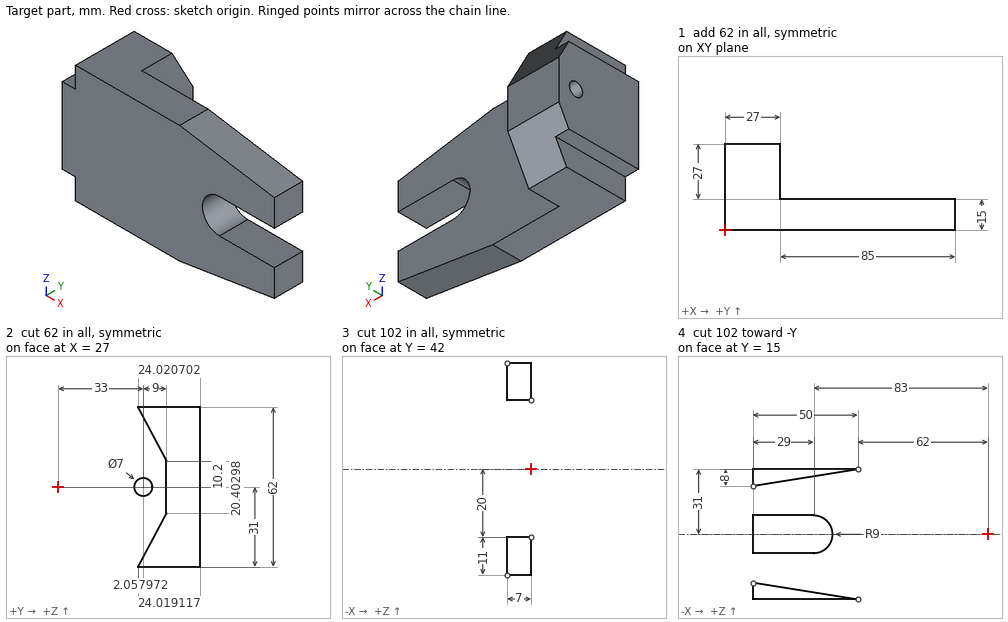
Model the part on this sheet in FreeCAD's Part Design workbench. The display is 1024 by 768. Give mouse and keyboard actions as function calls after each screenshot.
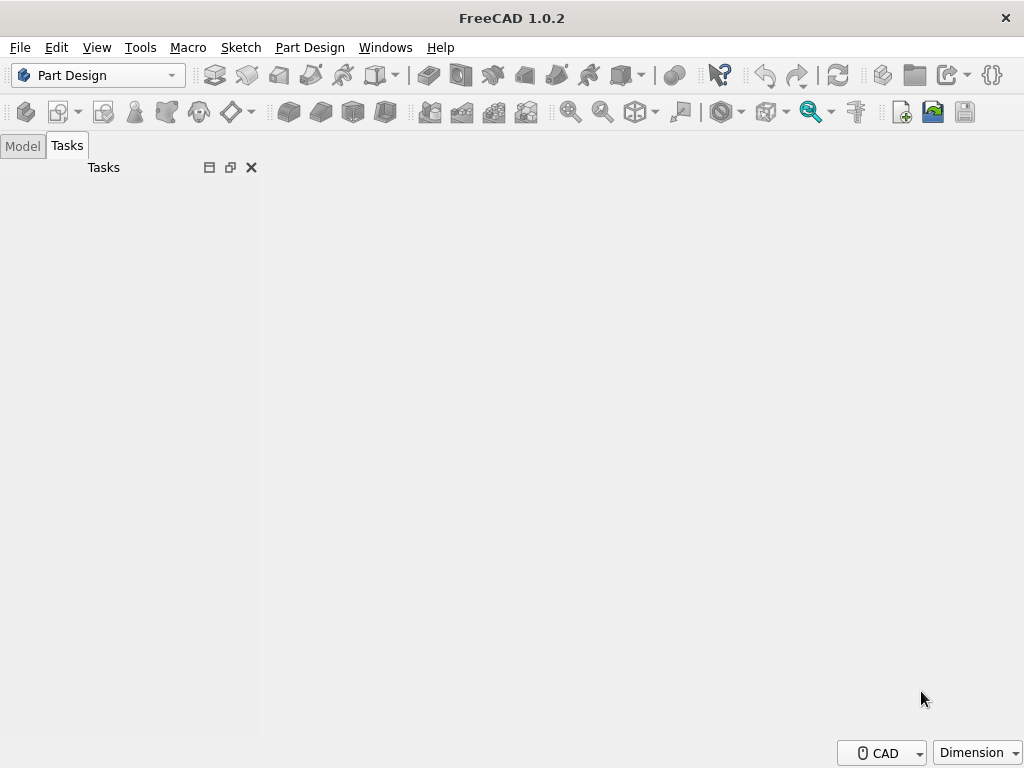
key(ctrl+n)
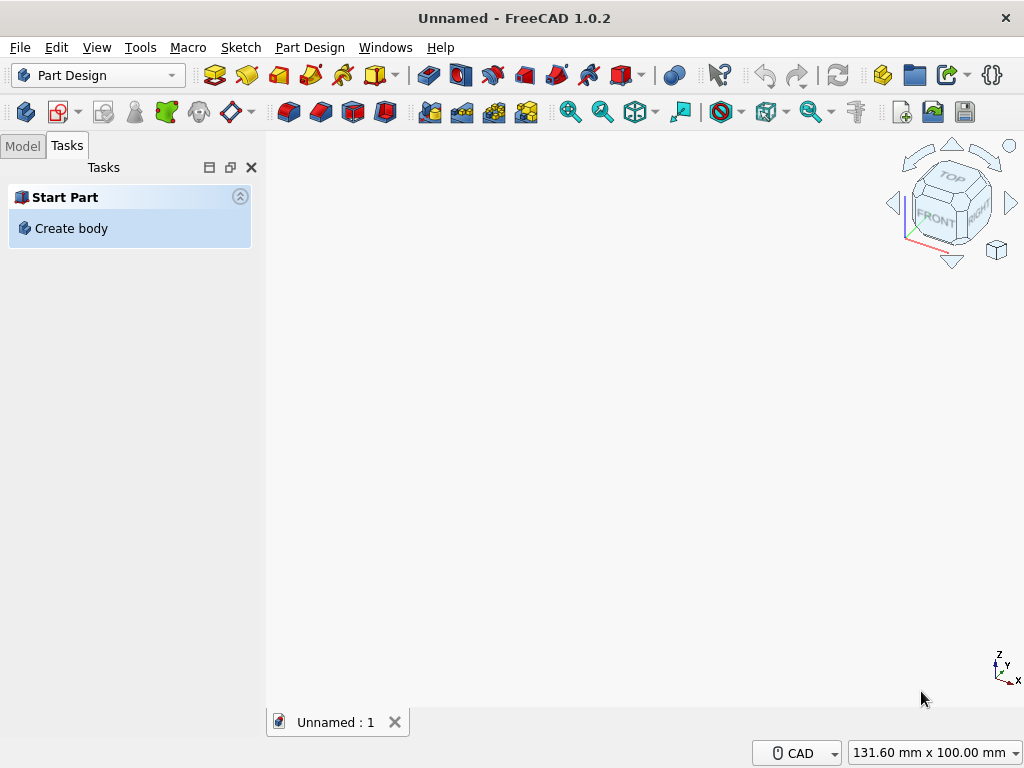
click(58, 112)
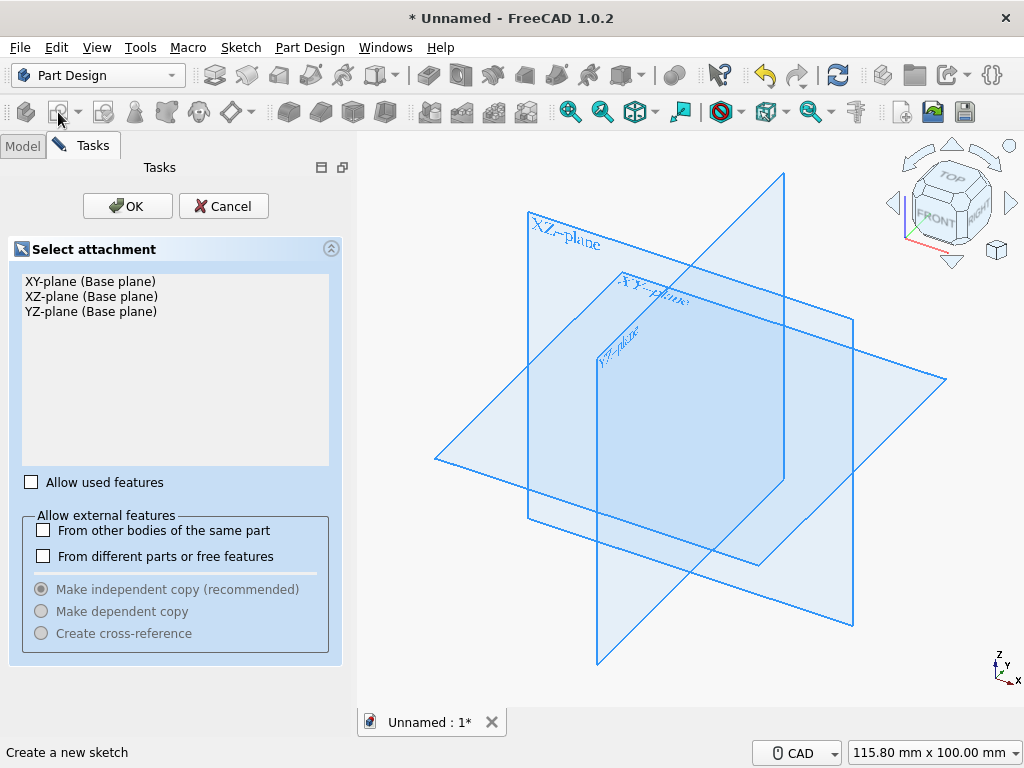
click(82, 282)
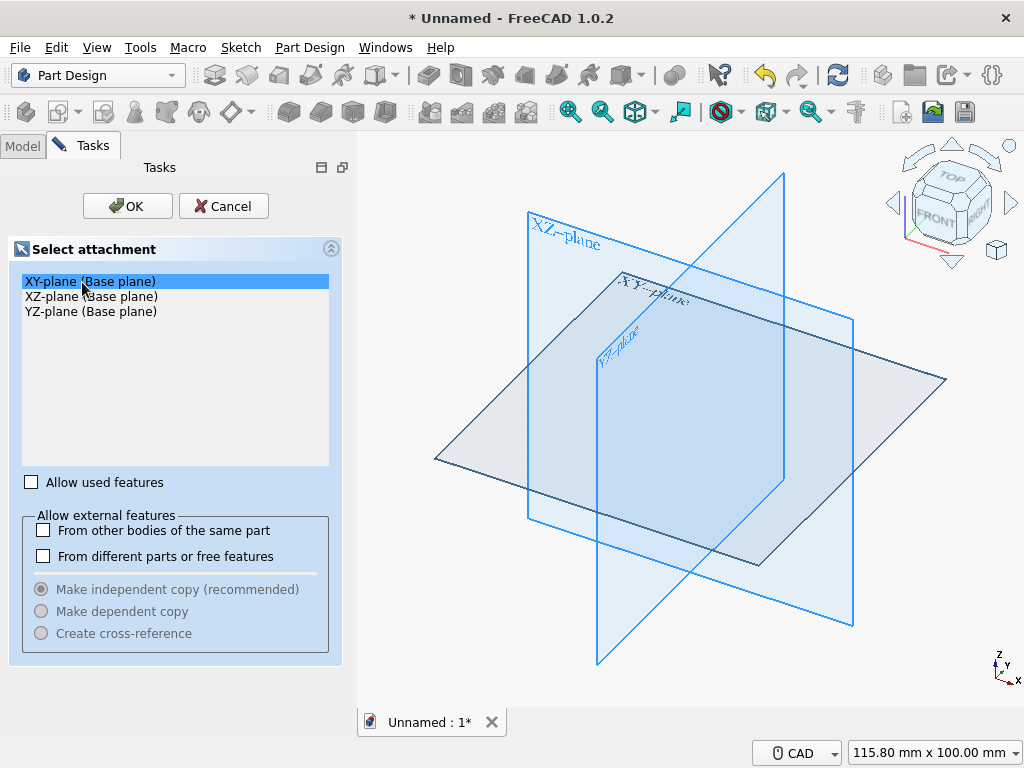
click(128, 206)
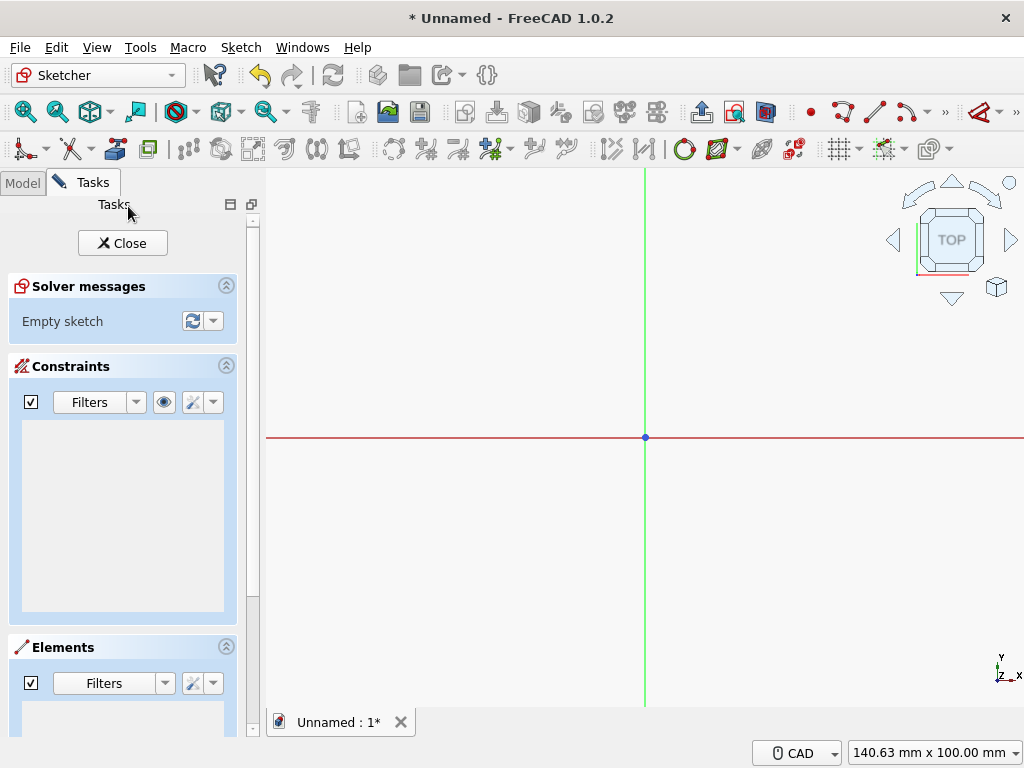
scroll(294, 575, down, 3)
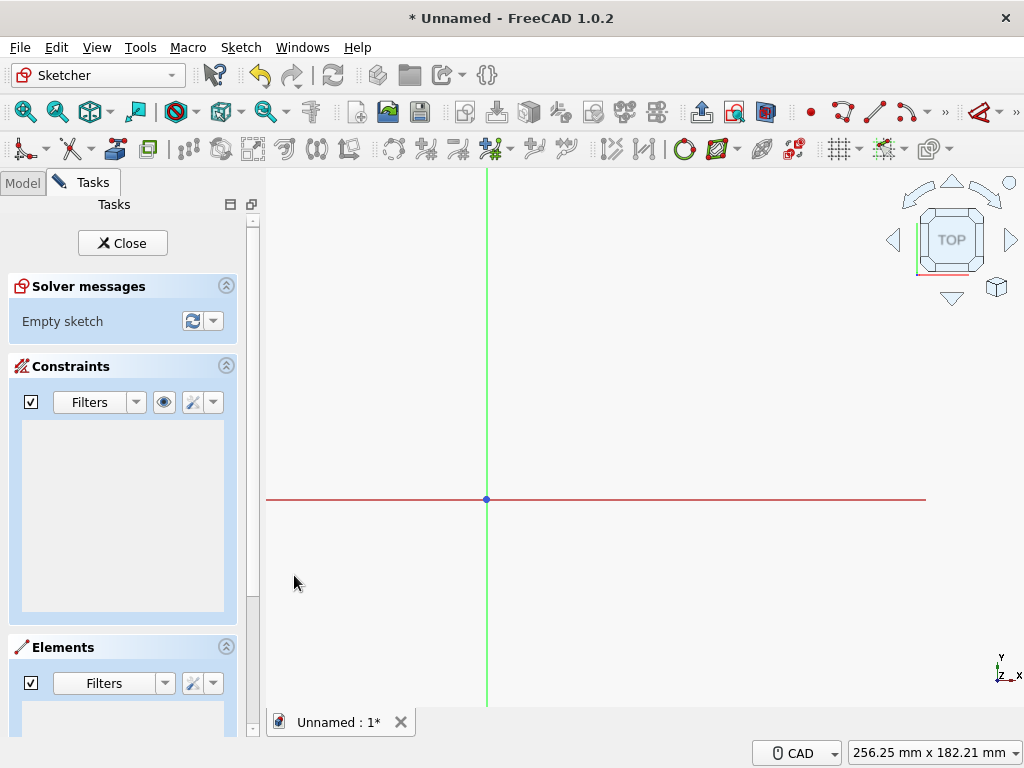
click(844, 112)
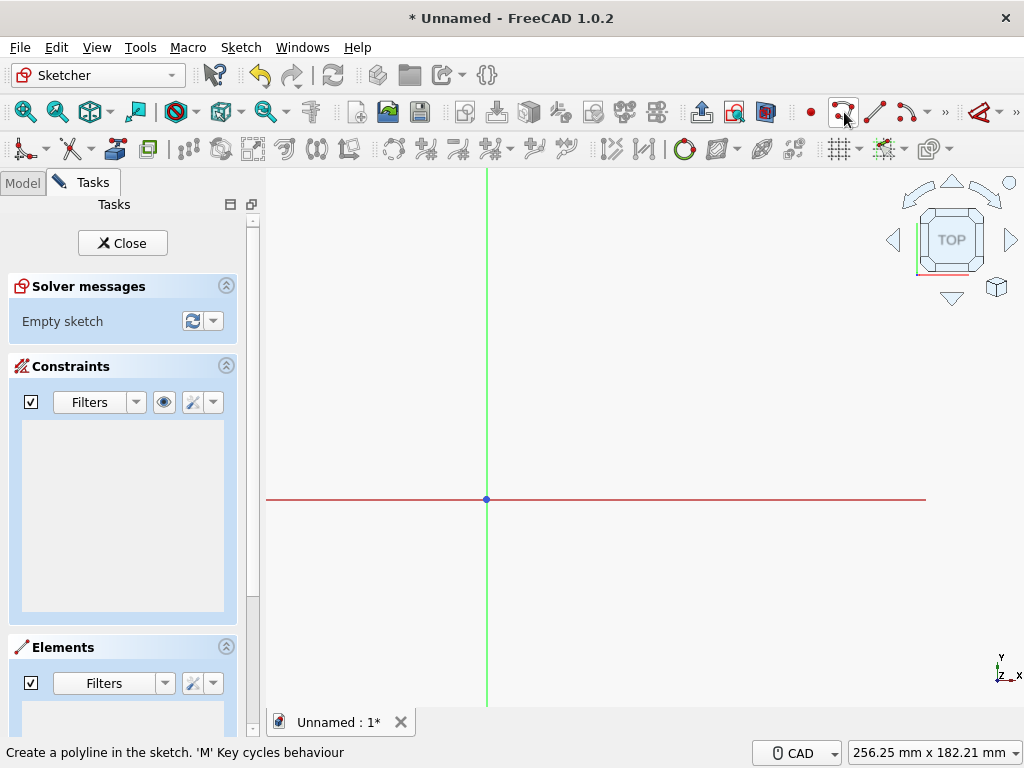
click(487, 500)
click(818, 491)
click(818, 456)
click(567, 456)
click(567, 376)
click(496, 376)
click(487, 500)
key(Escape)
key(Escape)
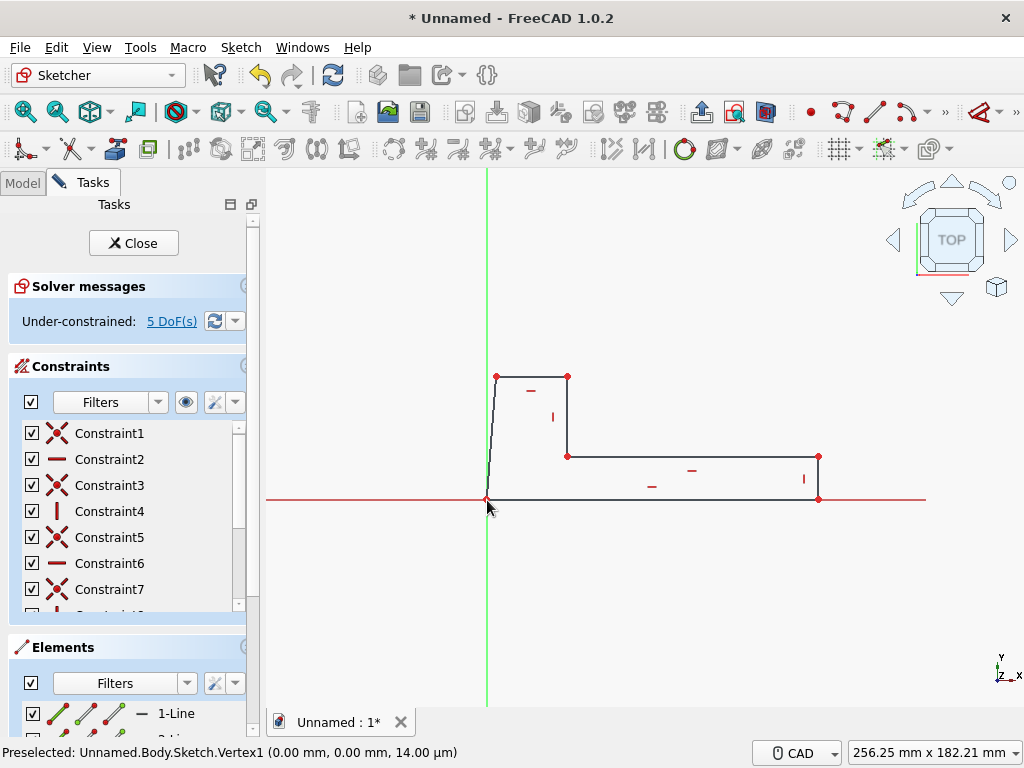
click(489, 463)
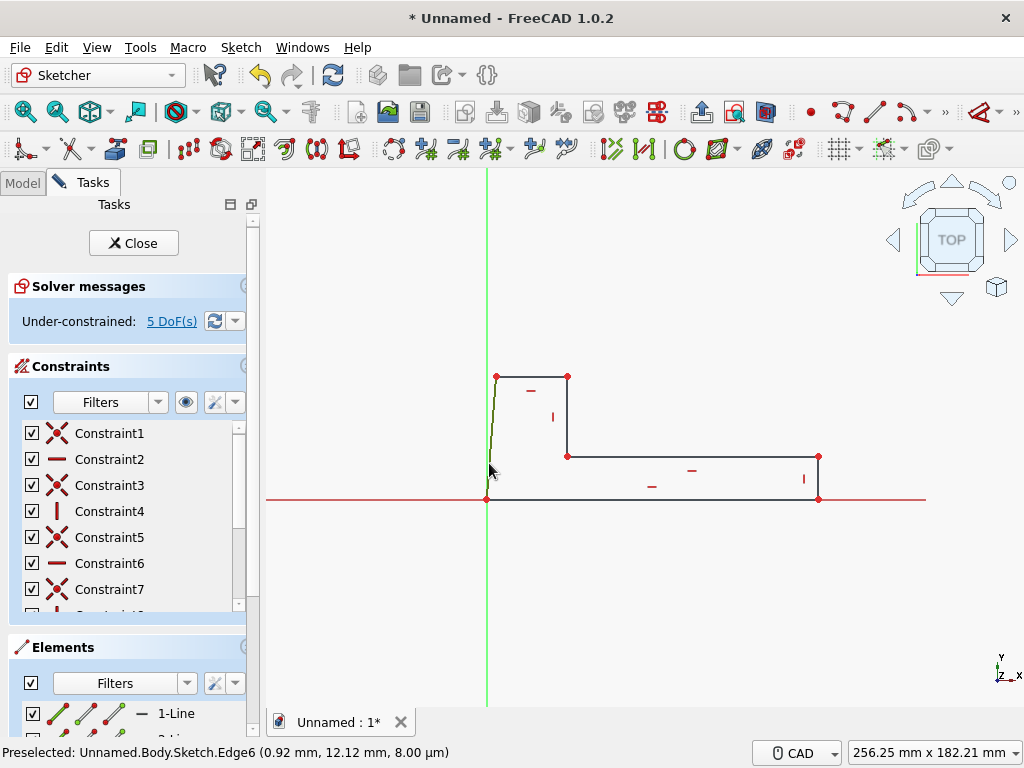
key(v)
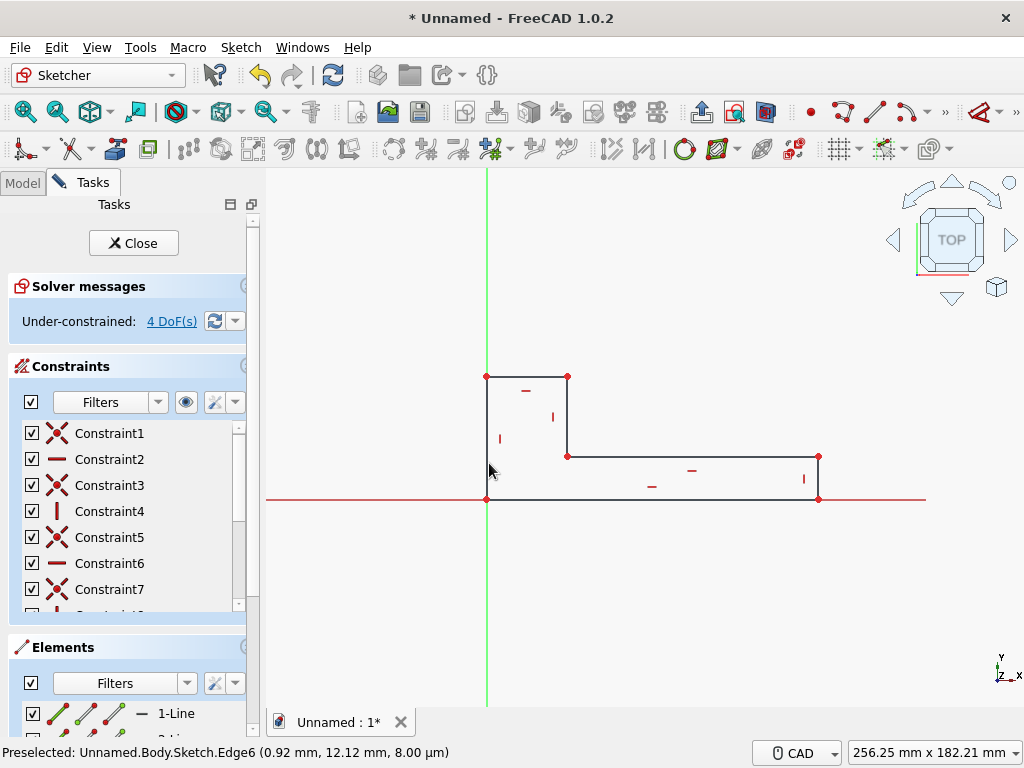
click(818, 487)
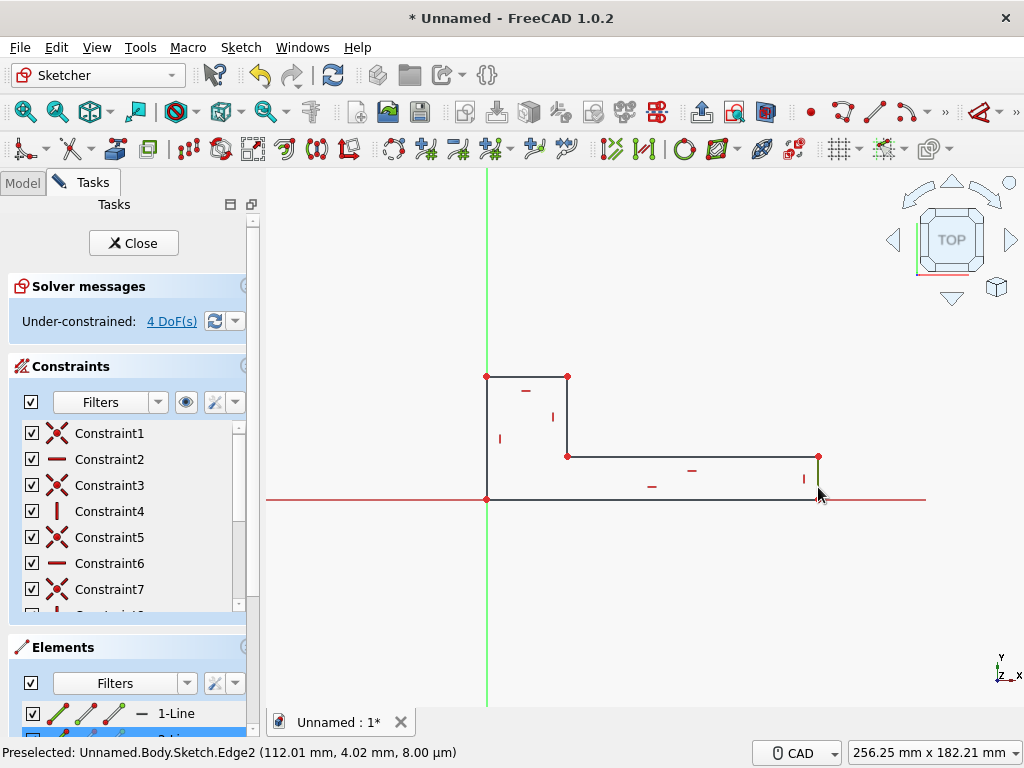
key(i)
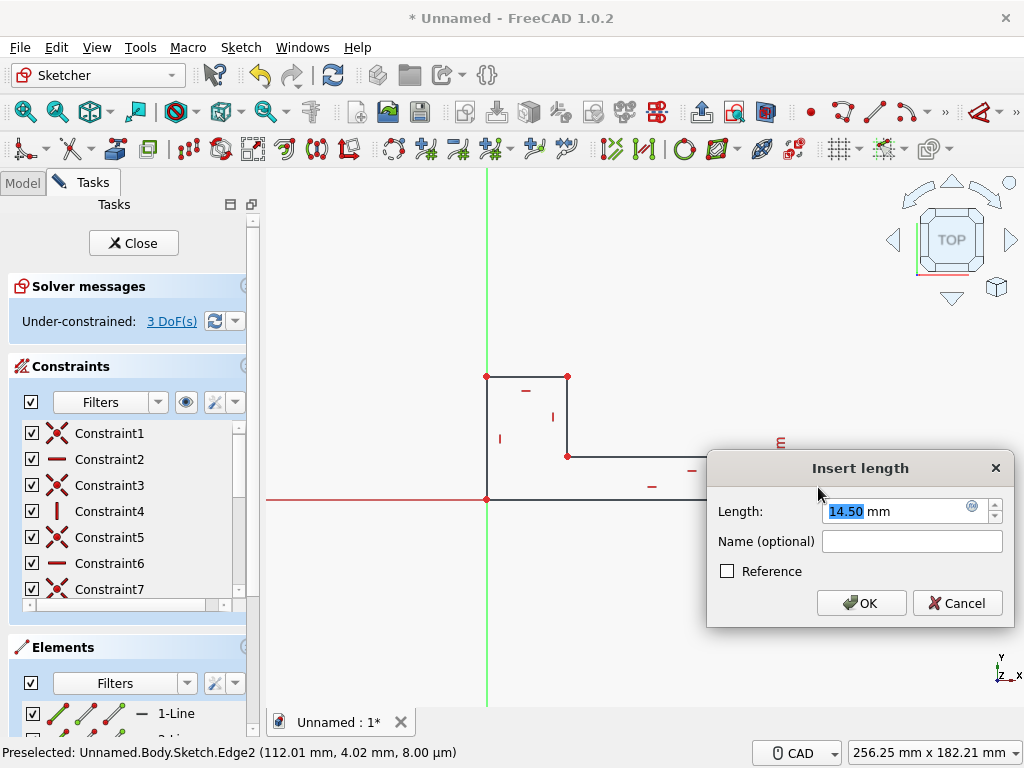
text(15)
key(Return)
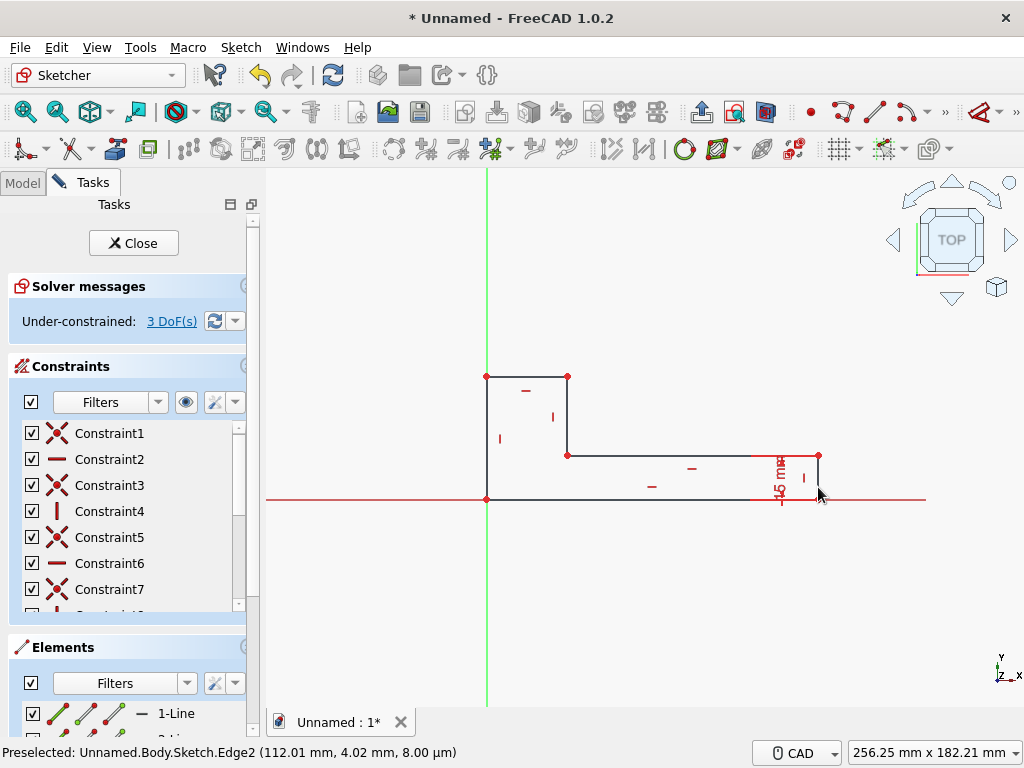
click(743, 456)